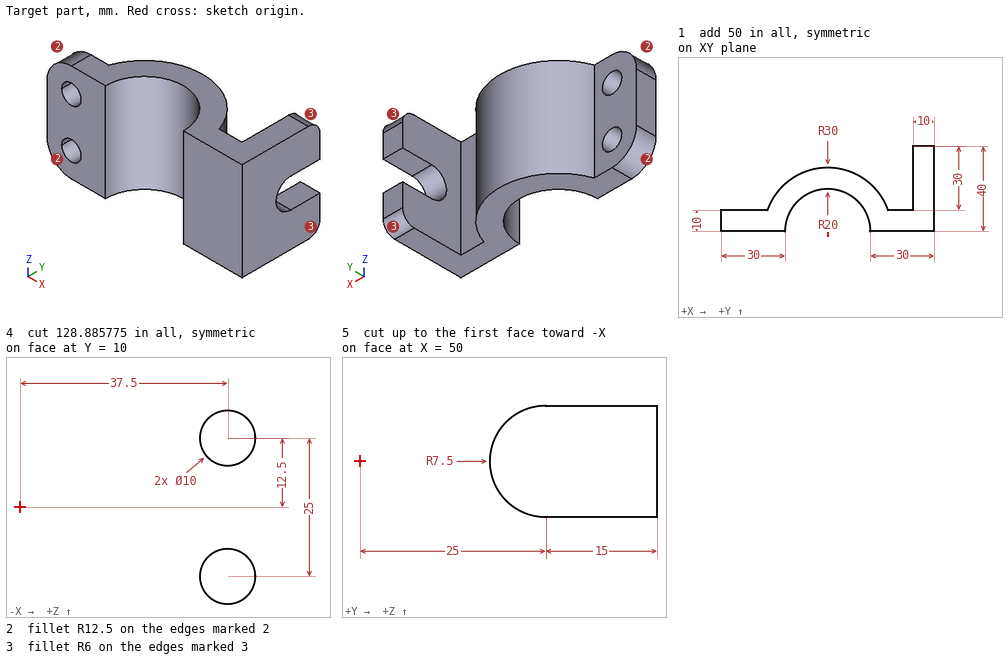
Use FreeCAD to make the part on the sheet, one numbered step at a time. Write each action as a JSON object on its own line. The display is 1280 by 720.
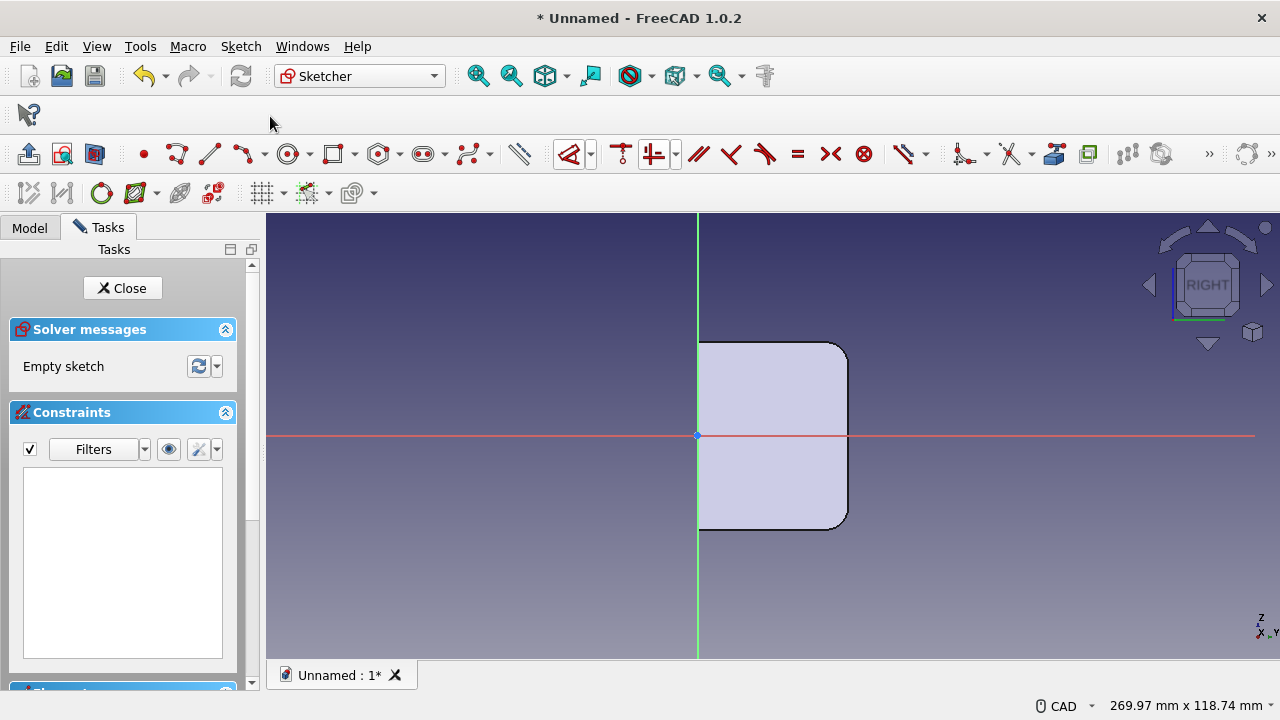
{"action": "scroll", "coordinate": [795, 436], "scroll_direction": "up", "scroll_amount": 7}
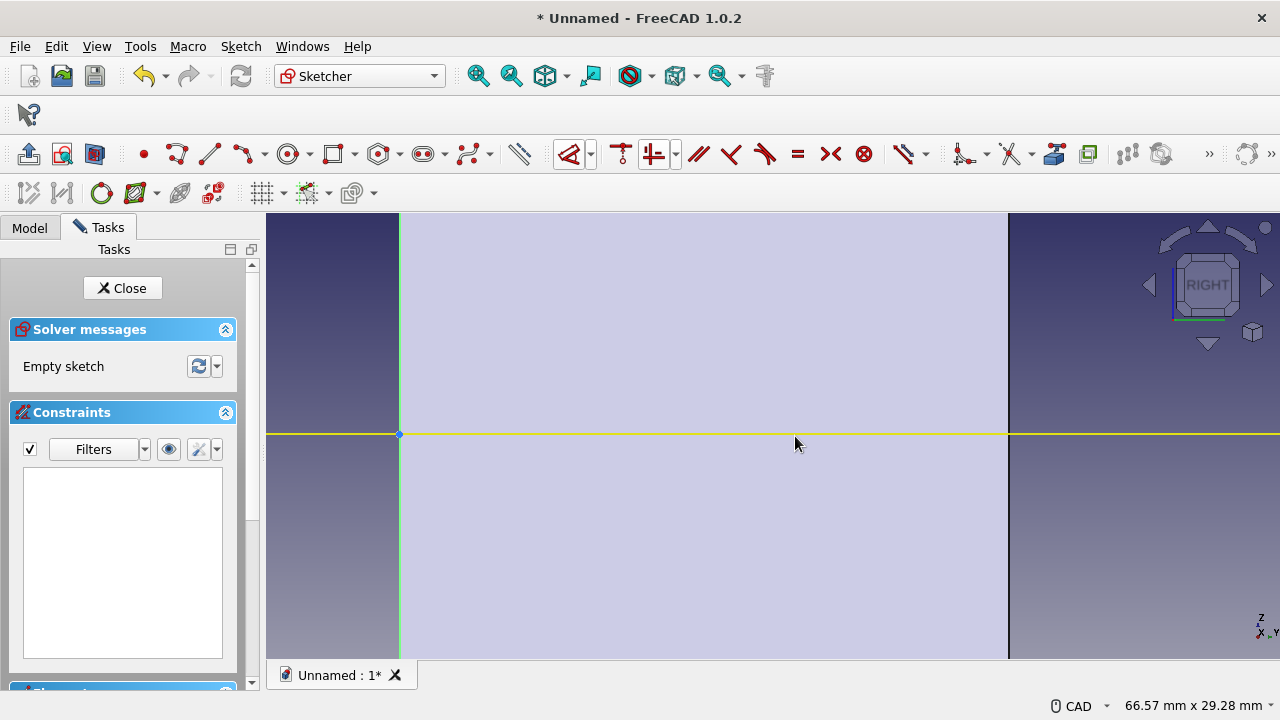
{"action": "left_click", "coordinate": [177, 154]}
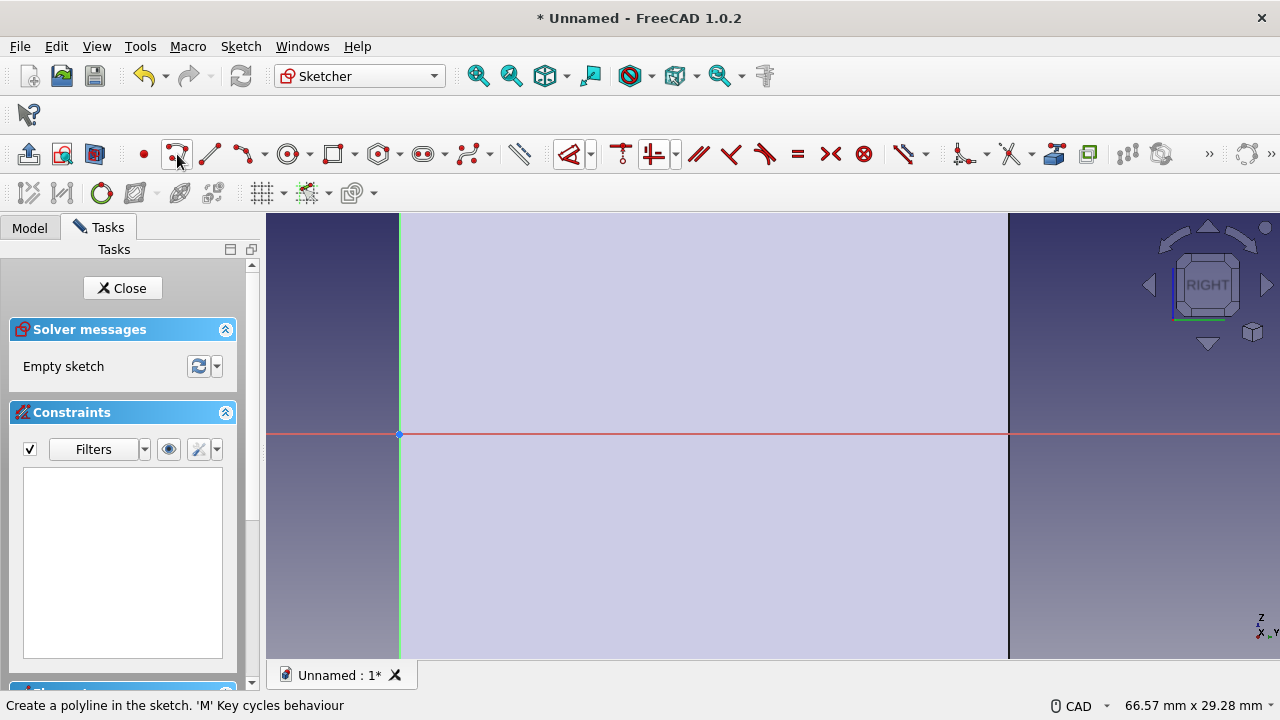
{"action": "left_click", "coordinate": [780, 549]}
{"action": "left_click", "coordinate": [1009, 549]}
{"action": "left_click", "coordinate": [1009, 320]}
{"action": "left_click", "coordinate": [780, 320]}
{"action": "right_click", "coordinate": [780, 320]}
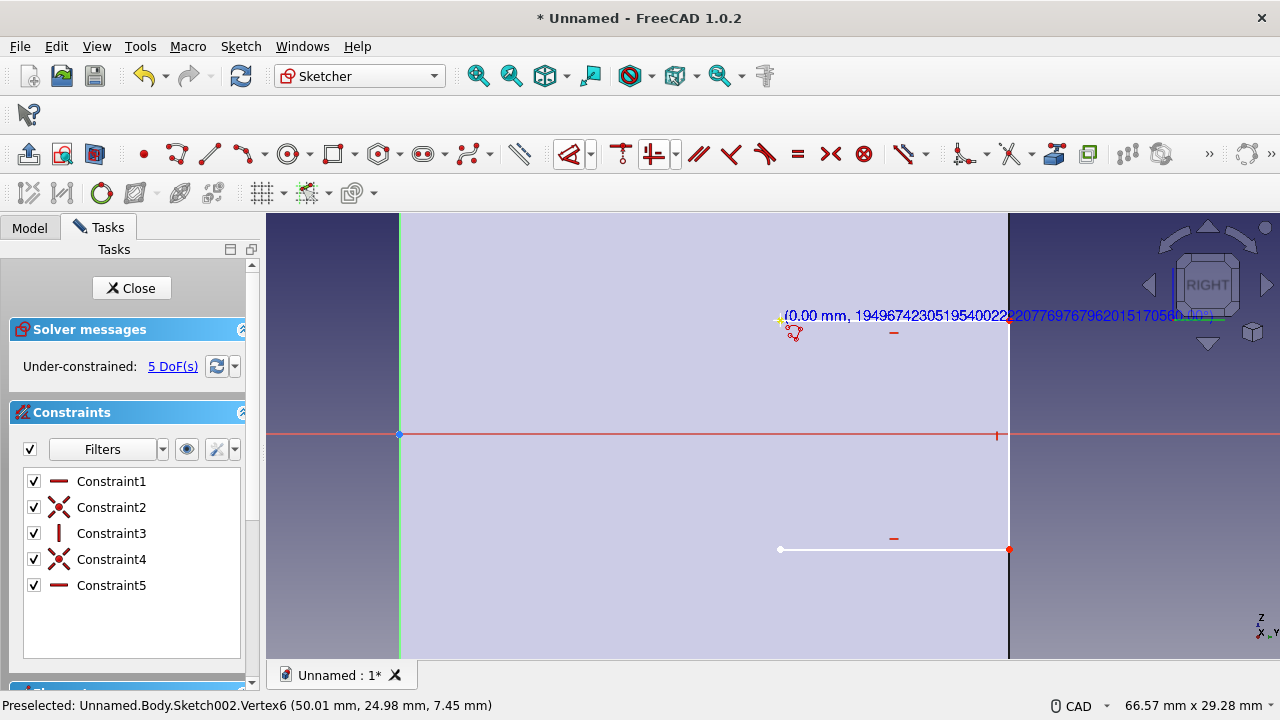
{"action": "left_click", "coordinate": [242, 154]}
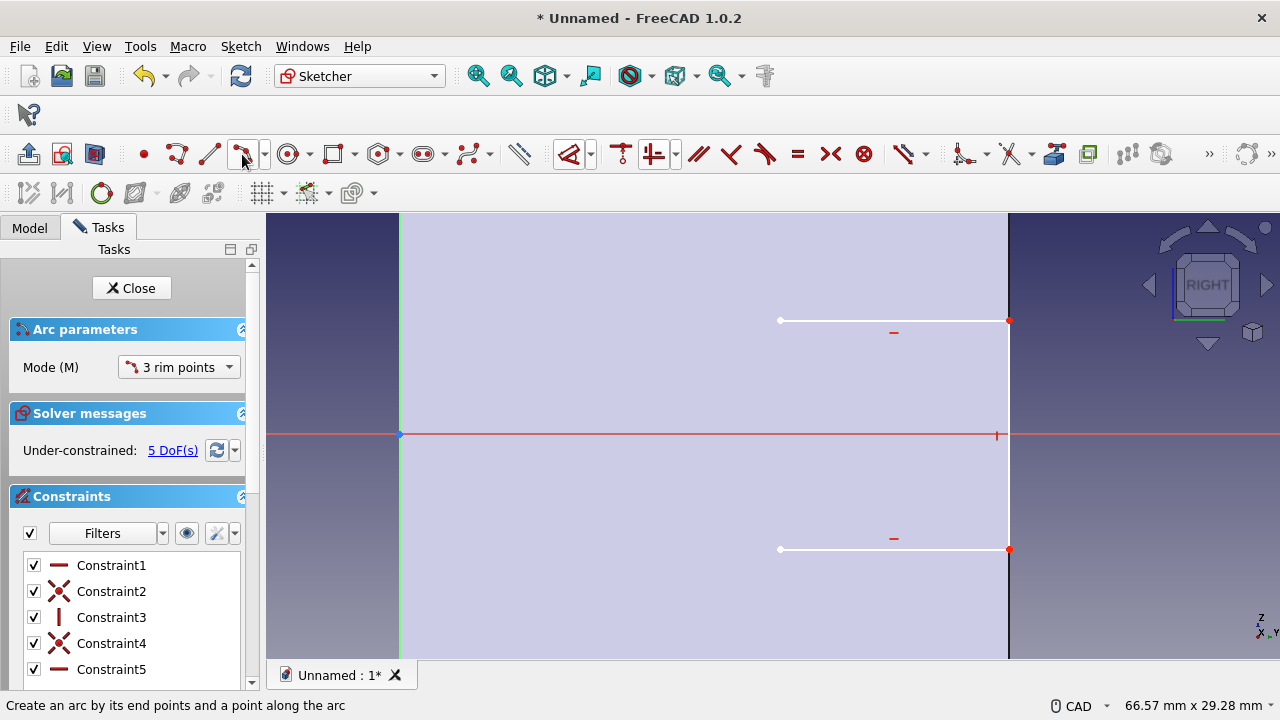
{"action": "left_click", "coordinate": [780, 321]}
{"action": "left_click", "coordinate": [780, 550]}
{"action": "left_click", "coordinate": [672, 399]}
{"action": "key", "text": "Escape"}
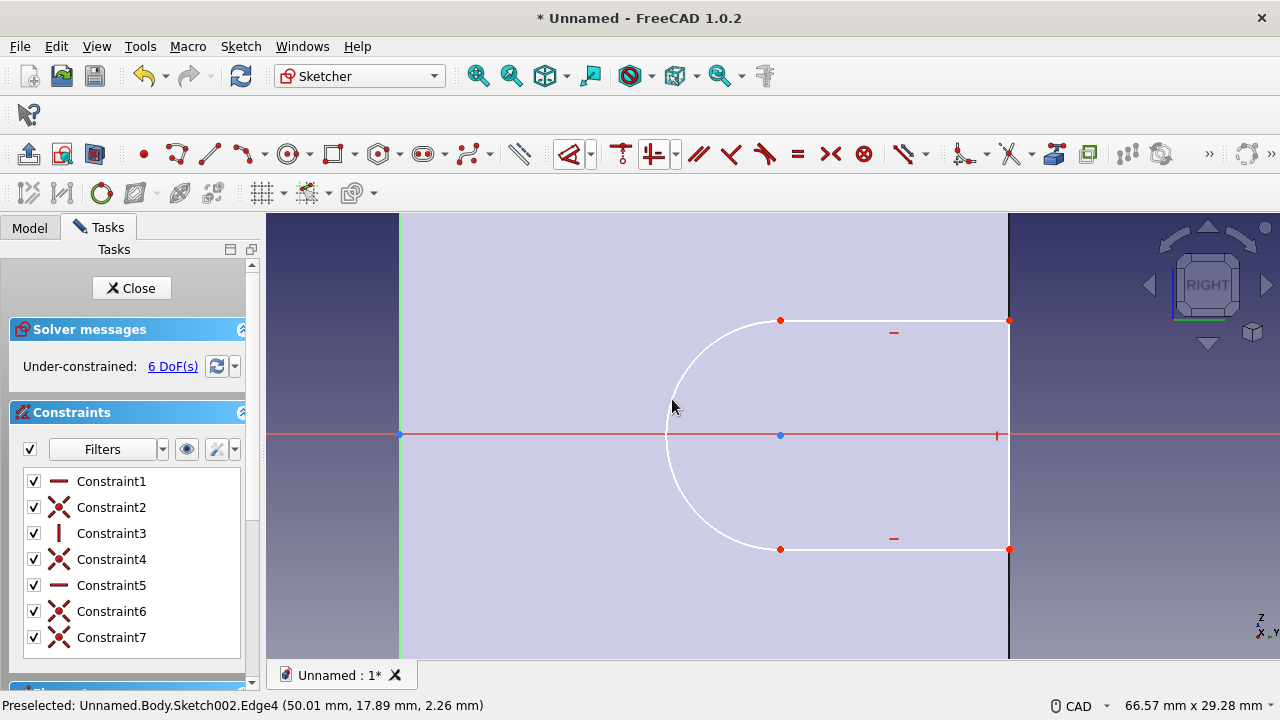
{"action": "left_click", "coordinate": [849, 550]}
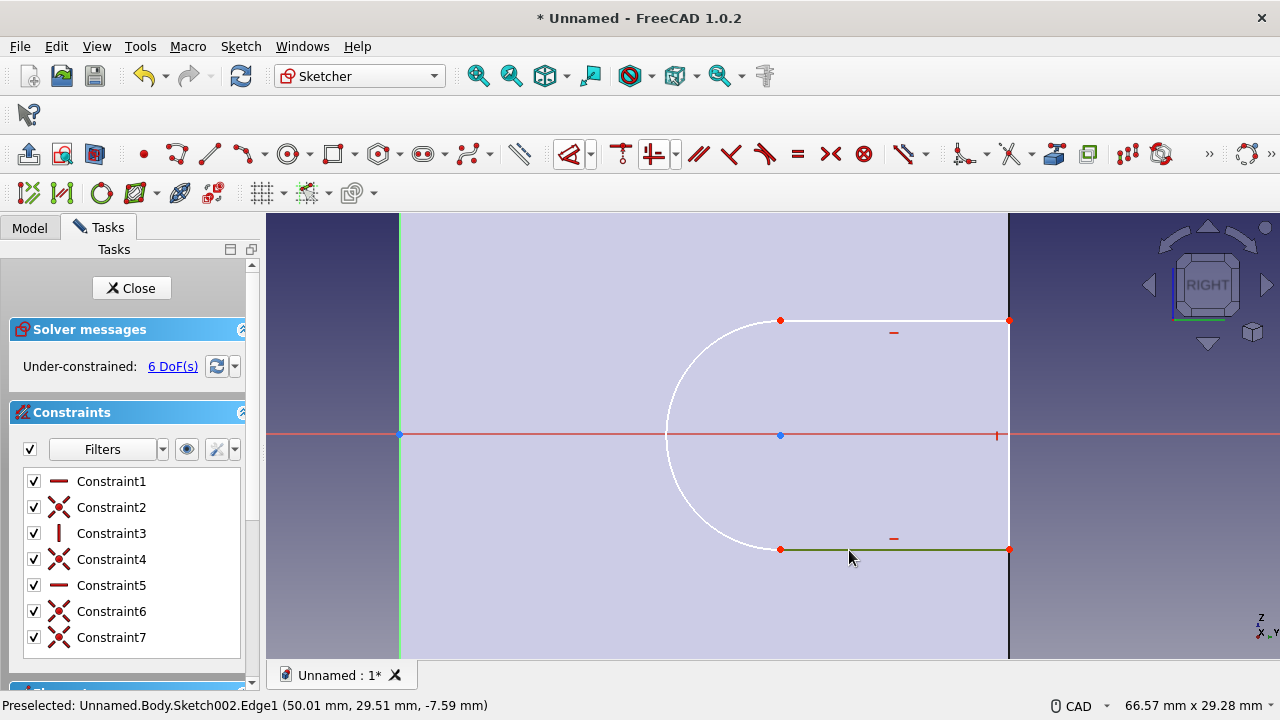
{"action": "left_click", "coordinate": [688, 368]}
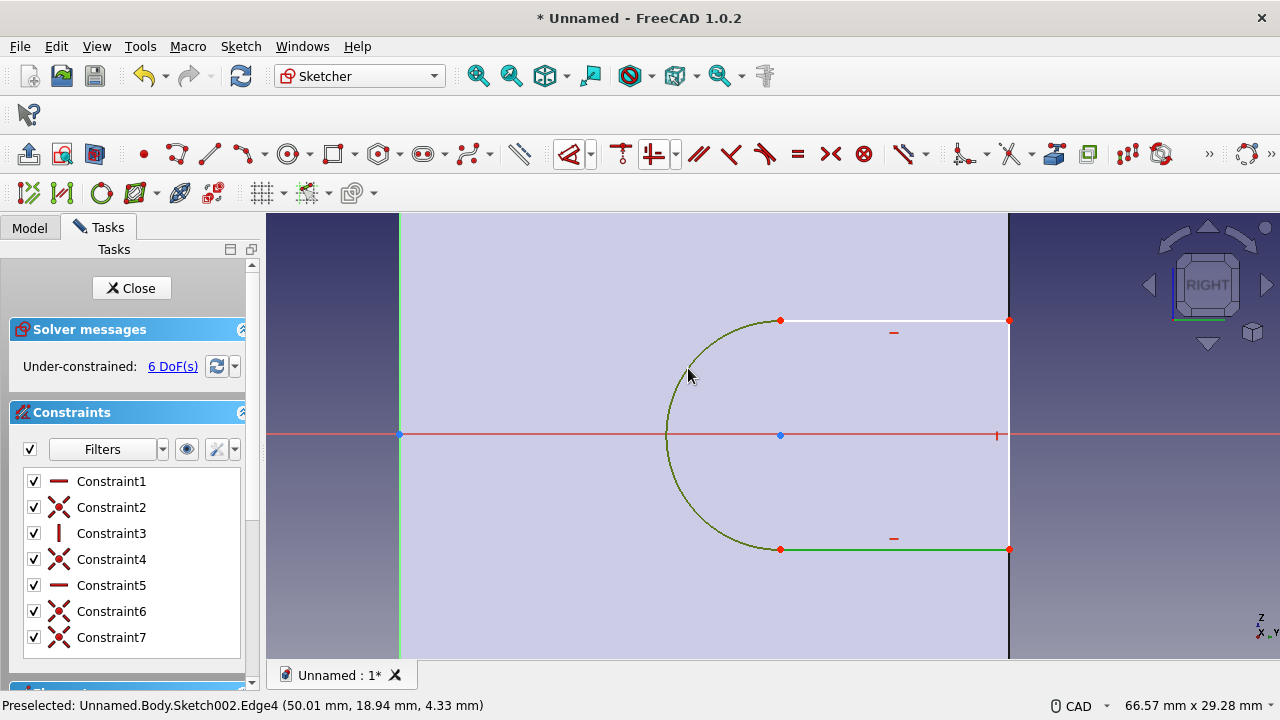
{"action": "left_click", "coordinate": [765, 154]}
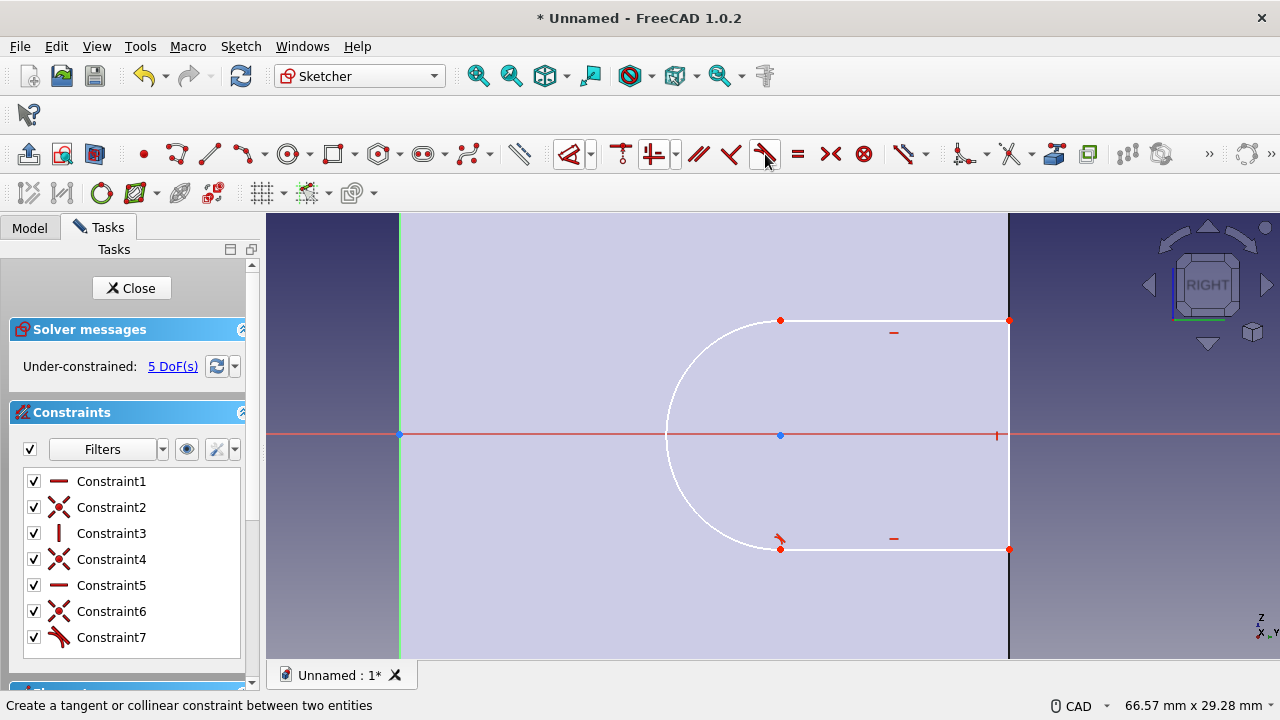
{"action": "left_click", "coordinate": [940, 321]}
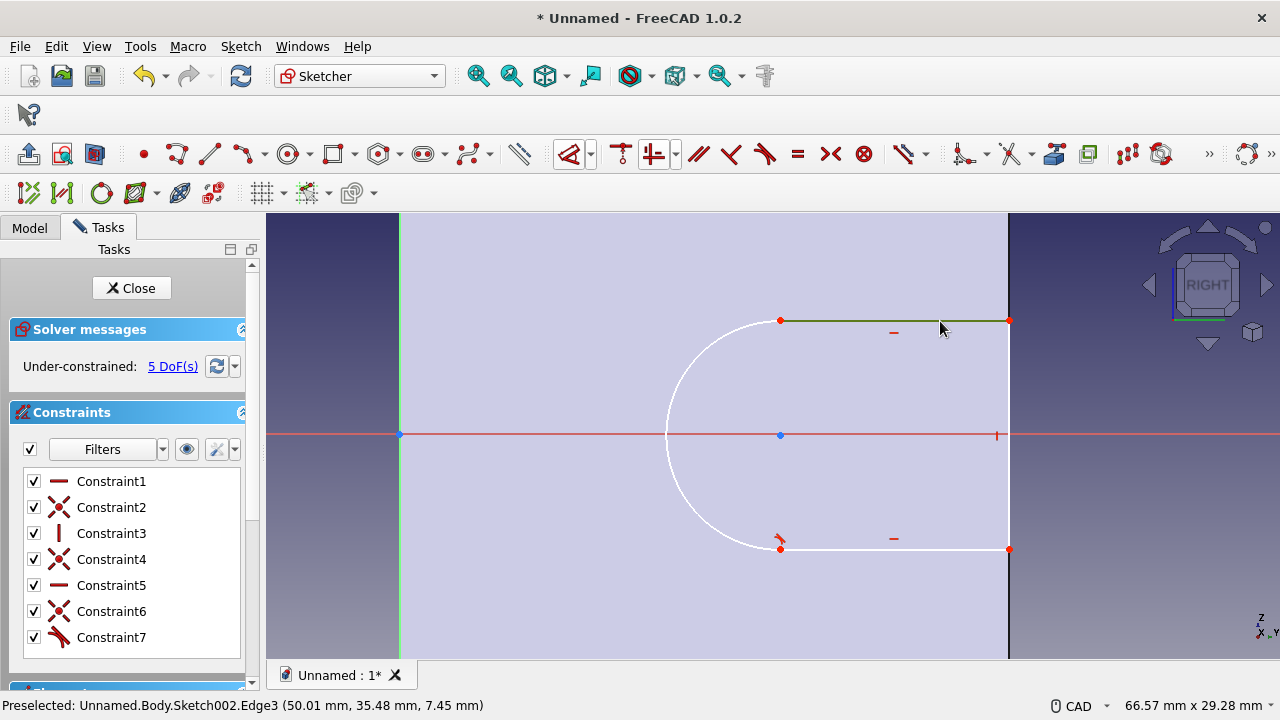
{"action": "left_click", "coordinate": [688, 369]}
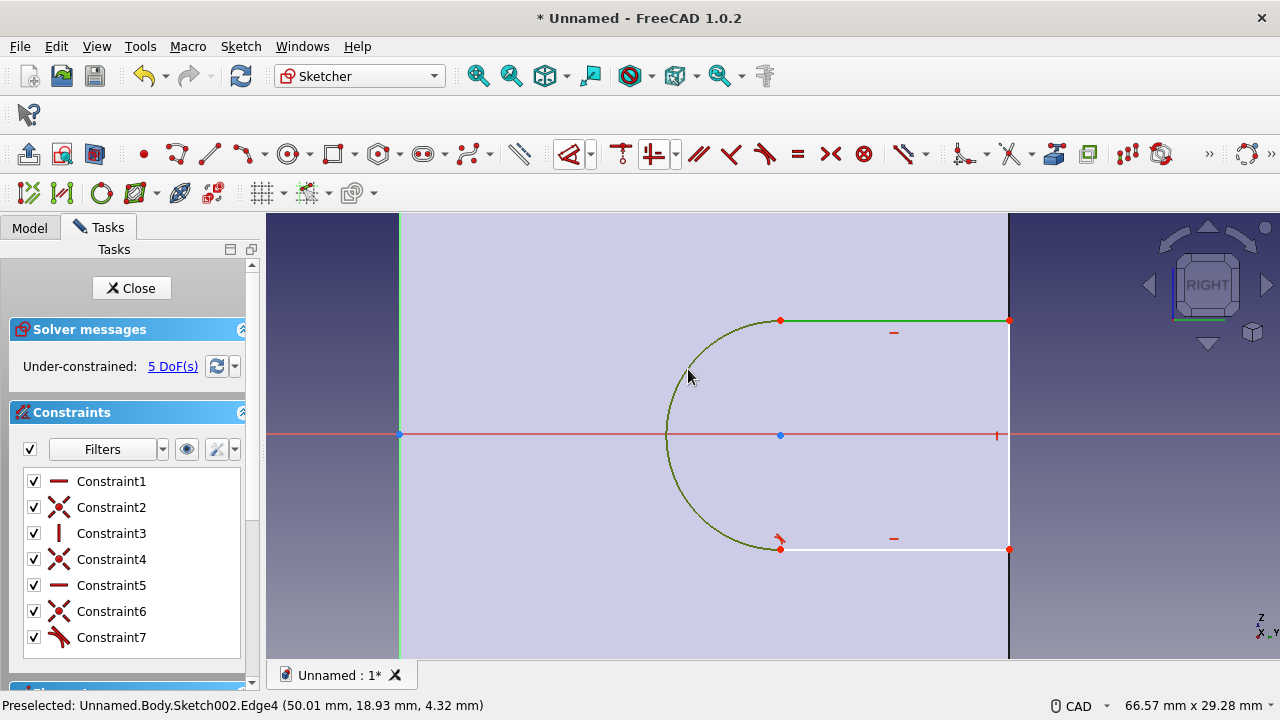
{"action": "left_click", "coordinate": [765, 154]}